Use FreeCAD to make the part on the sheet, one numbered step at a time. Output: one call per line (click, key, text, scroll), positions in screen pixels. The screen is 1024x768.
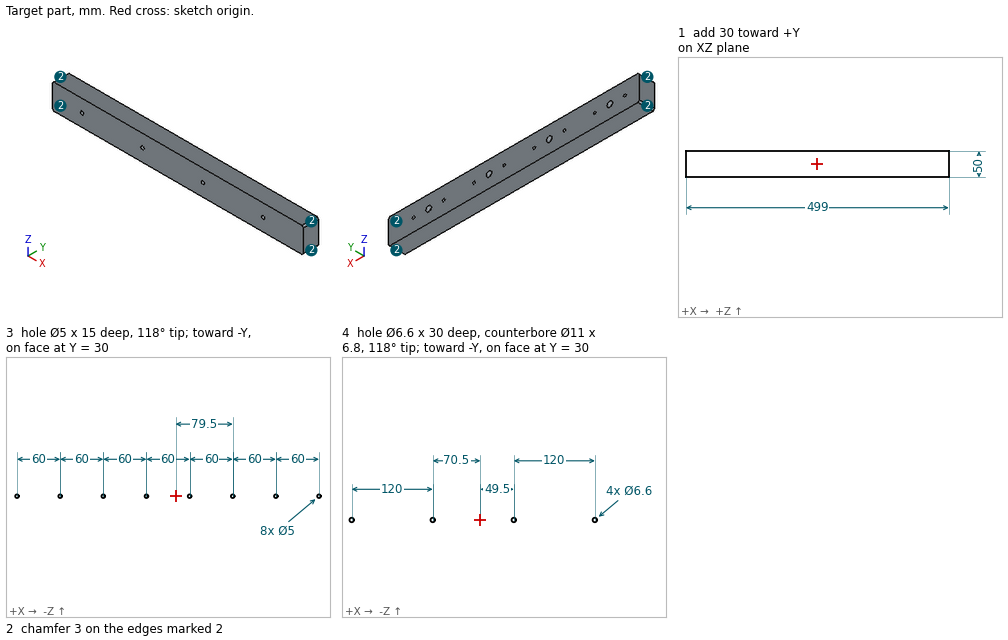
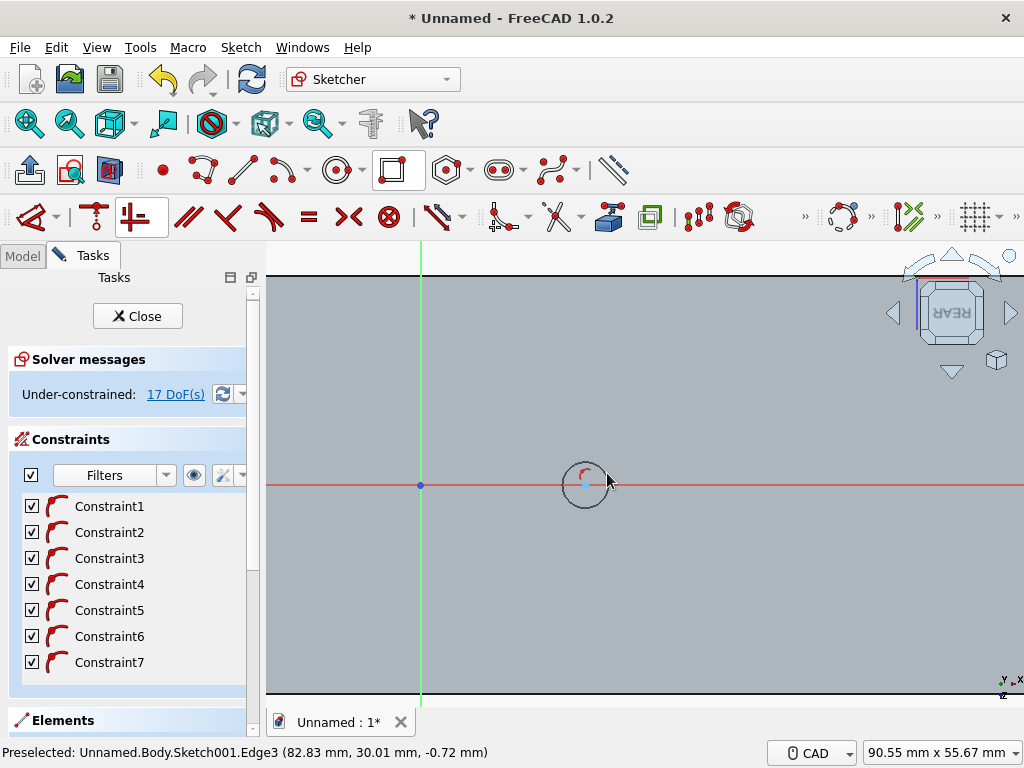
click(601, 469)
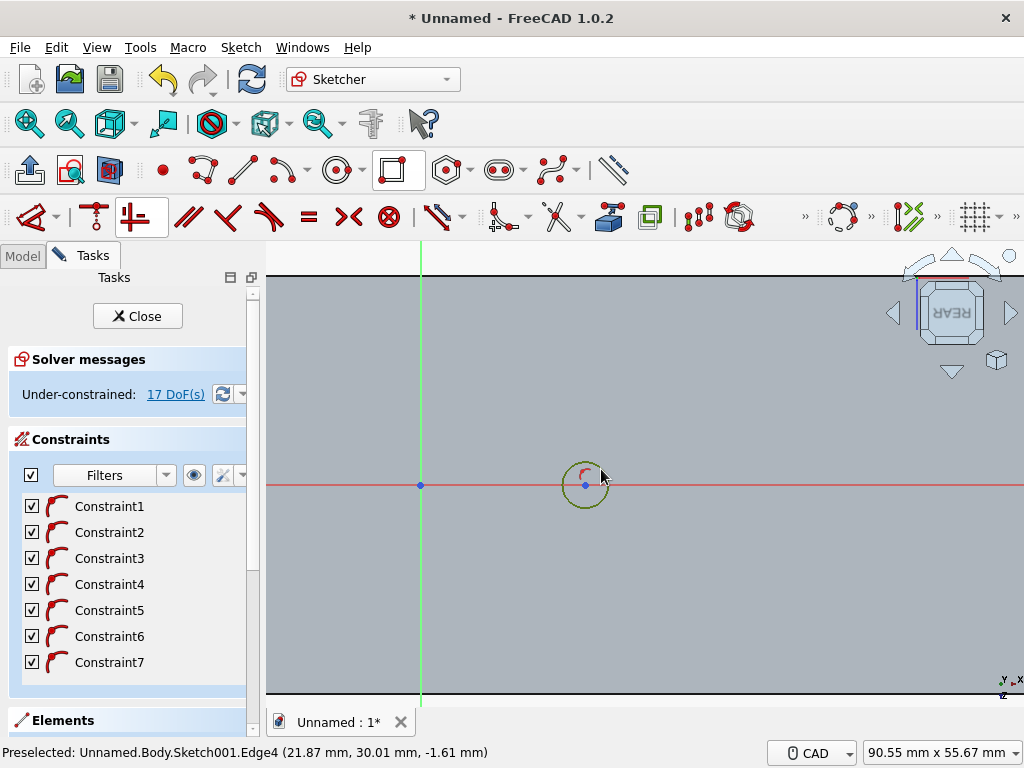
scroll(607, 473, down, 11)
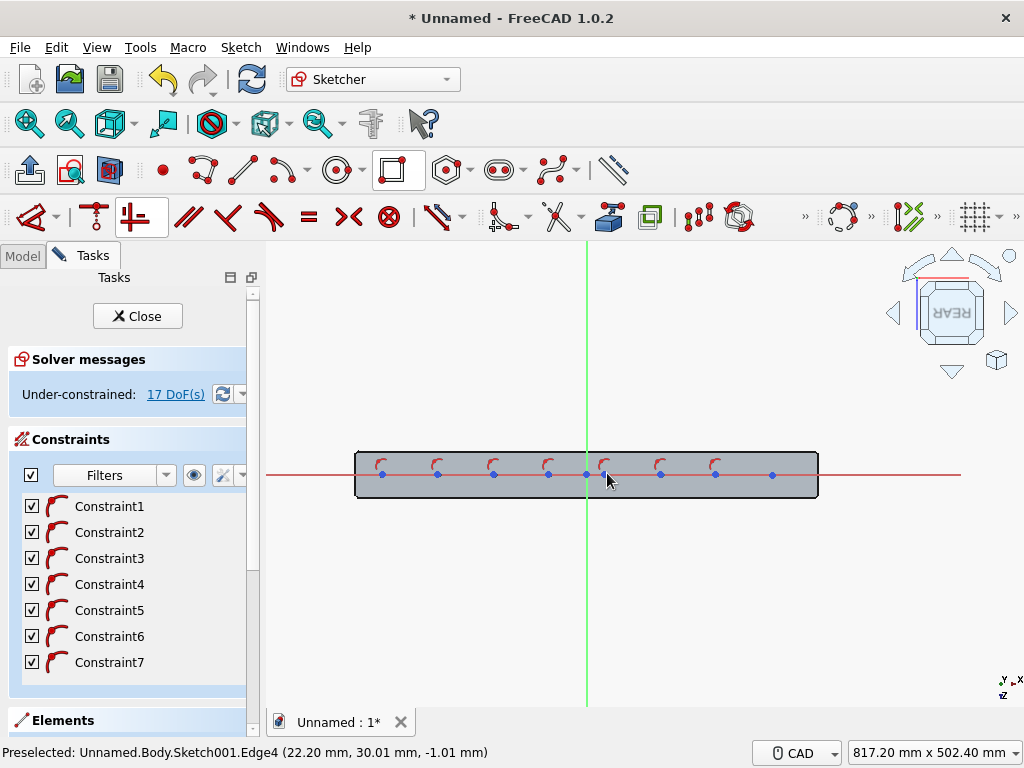
scroll(551, 473, up, 11)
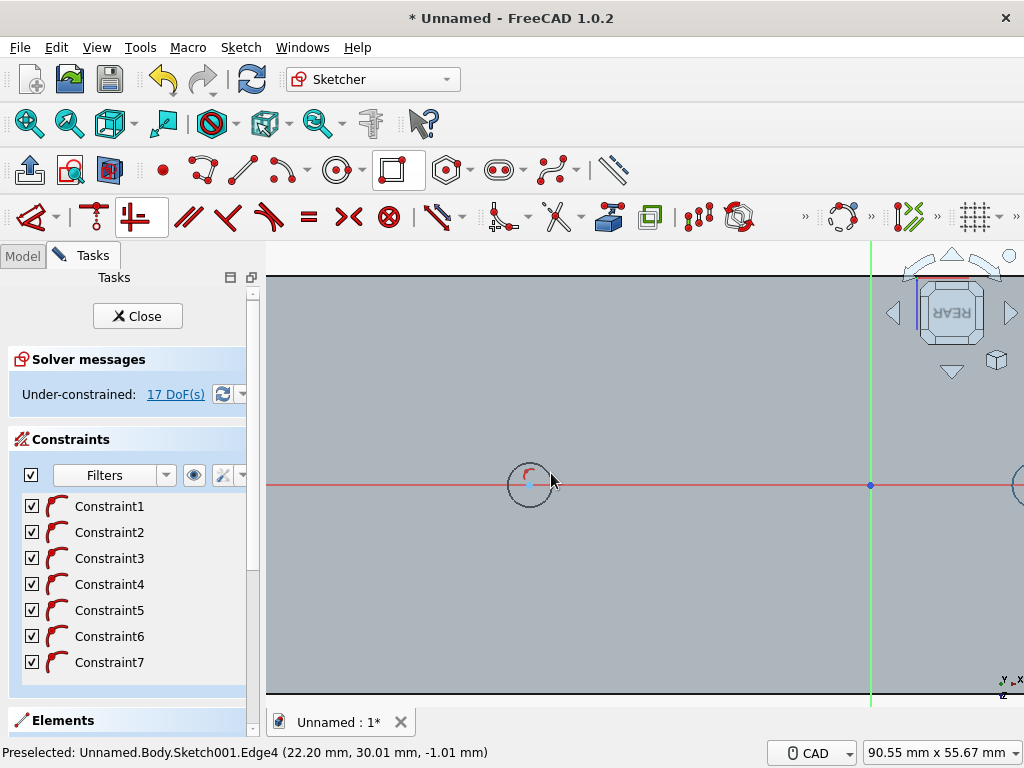
click(545, 470)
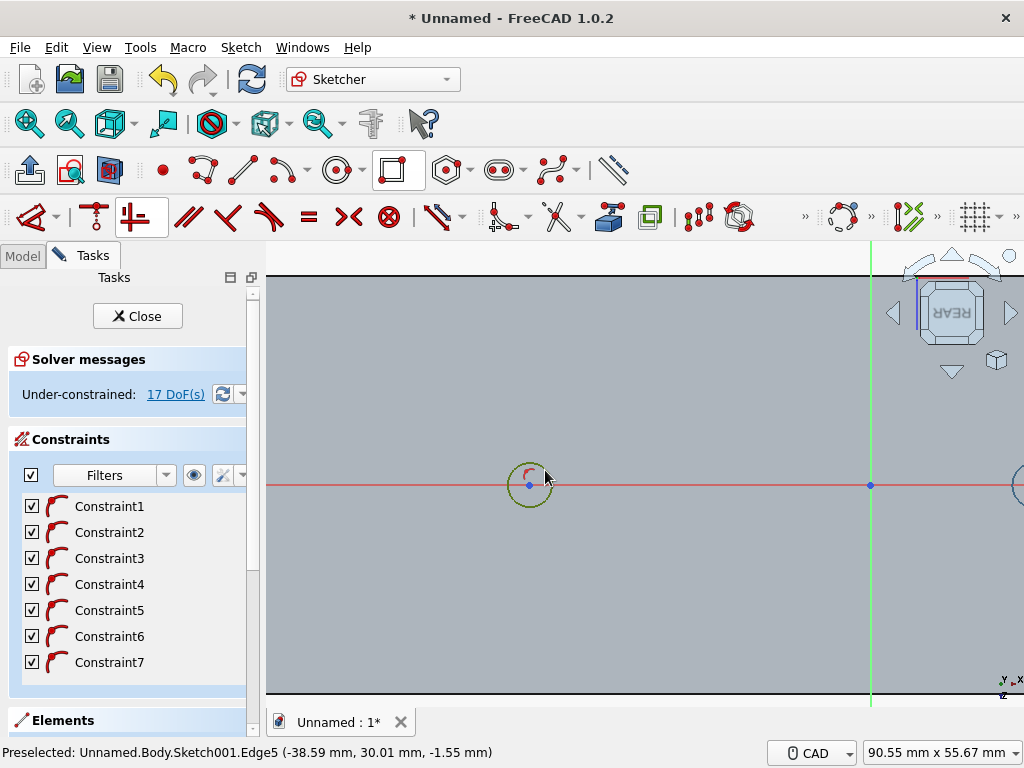
scroll(551, 473, down, 11)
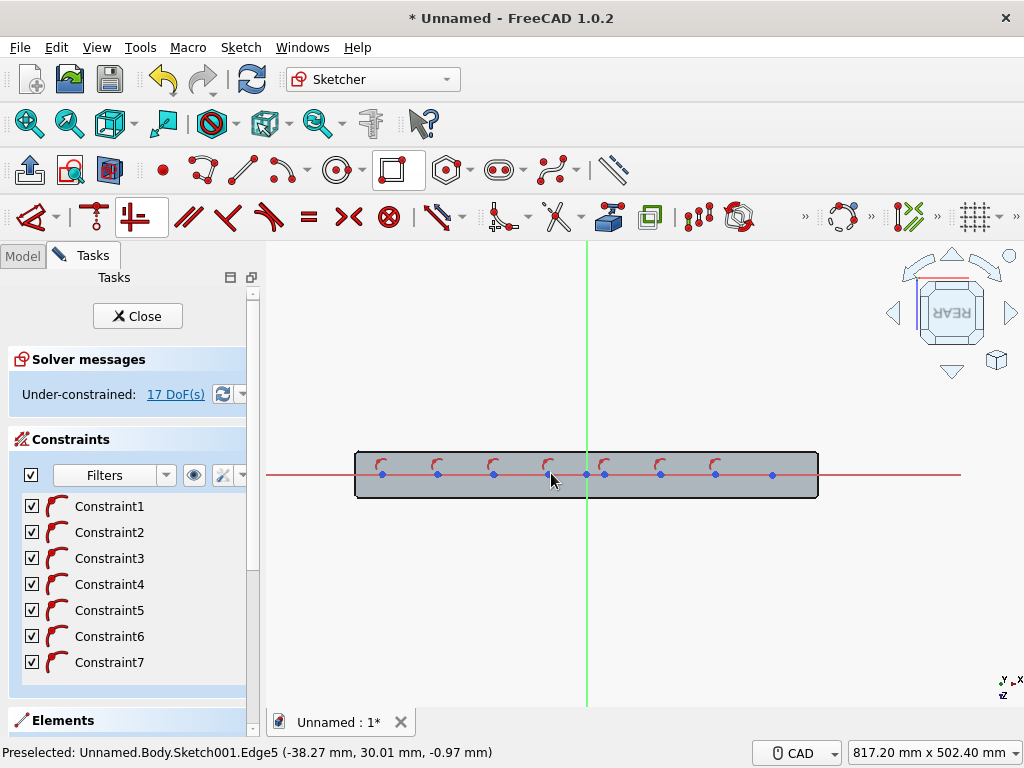
scroll(496, 473, up, 10)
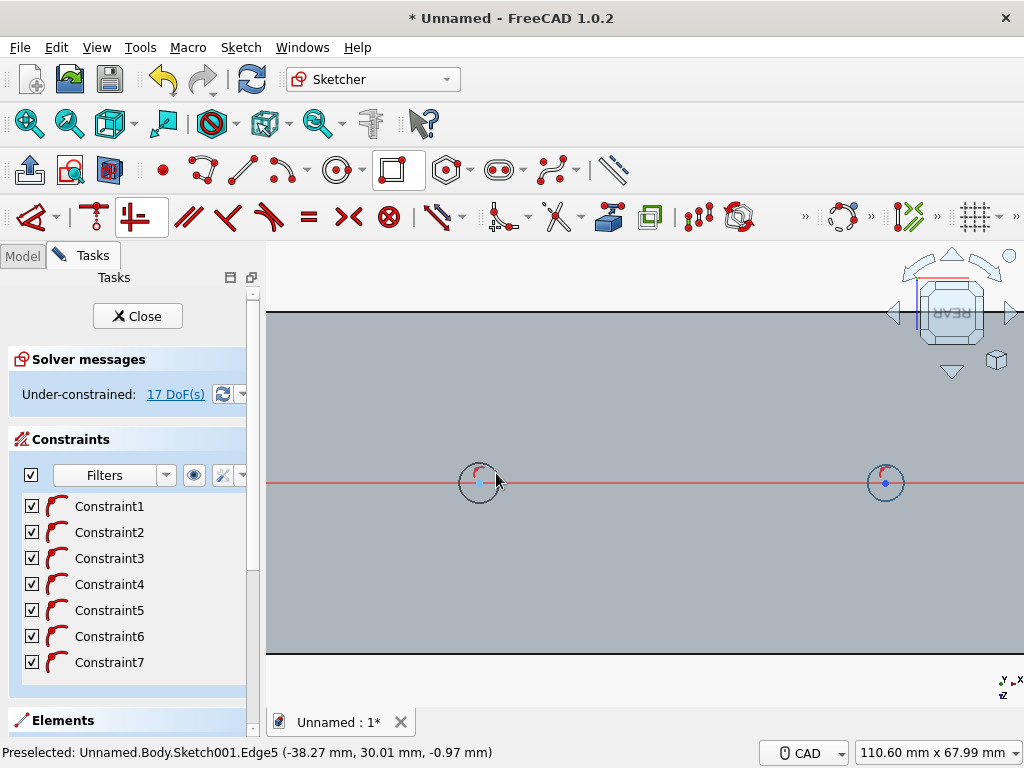
click(493, 469)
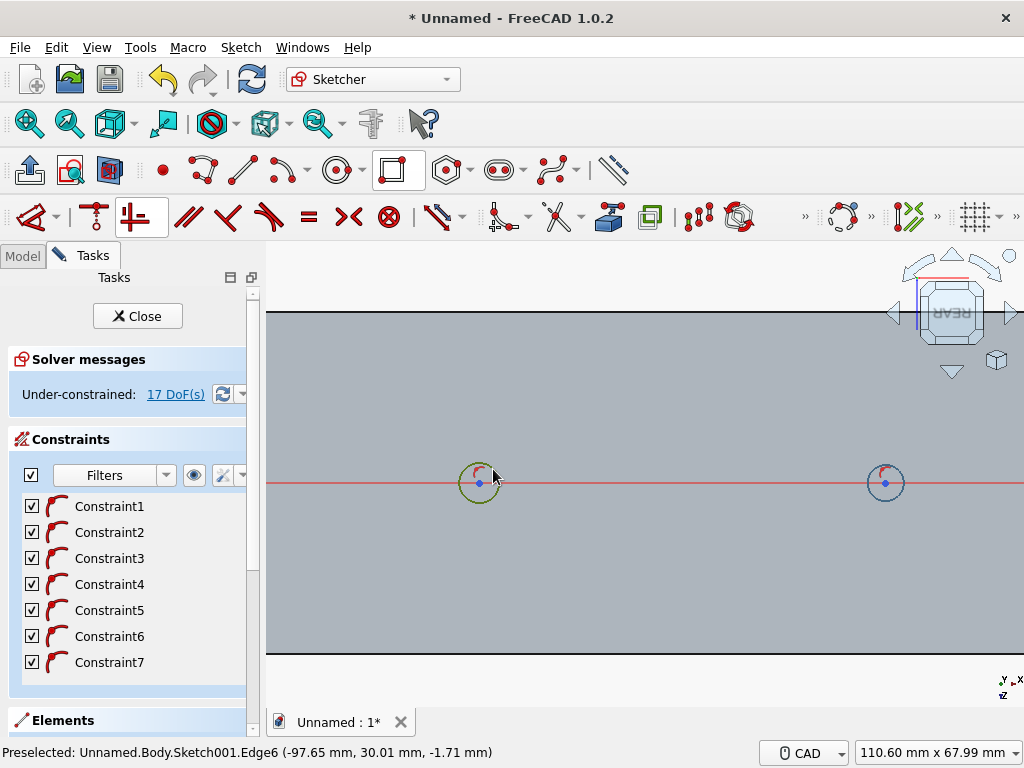
scroll(496, 473, down, 10)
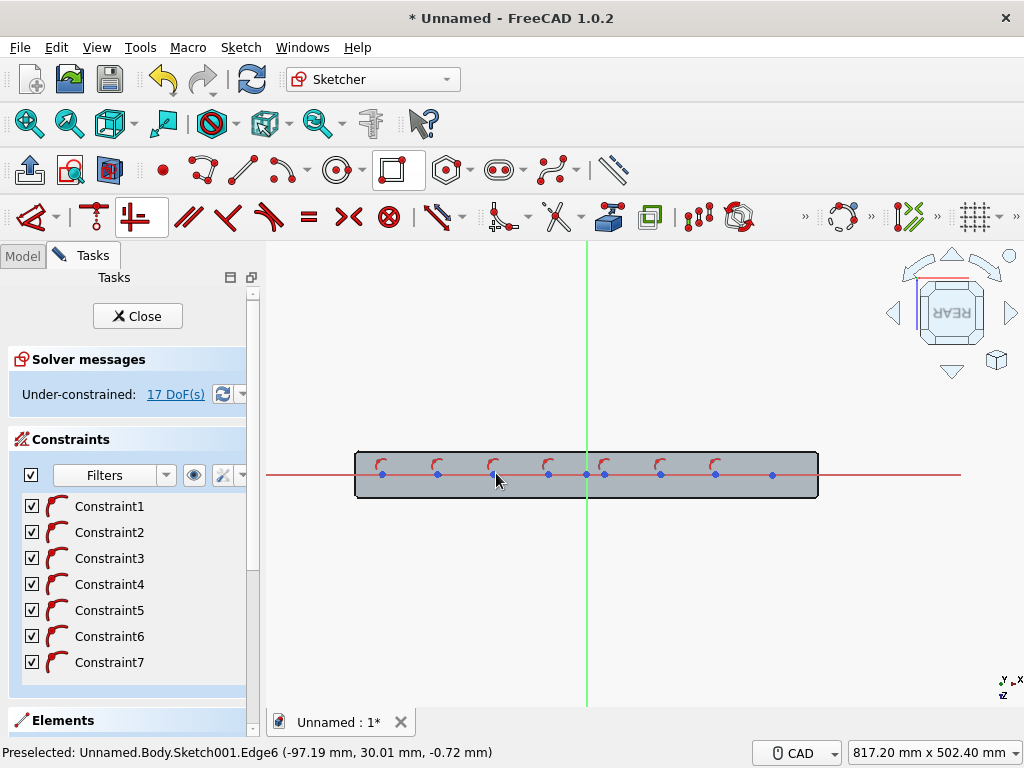
scroll(440, 473, up, 11)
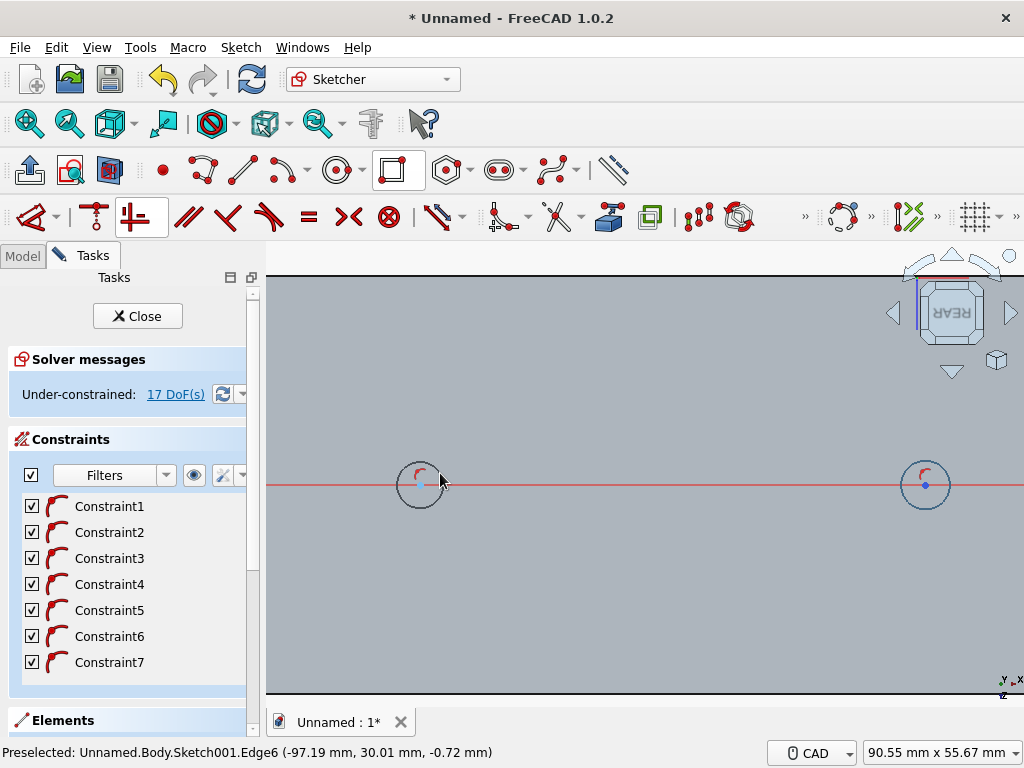
click(436, 469)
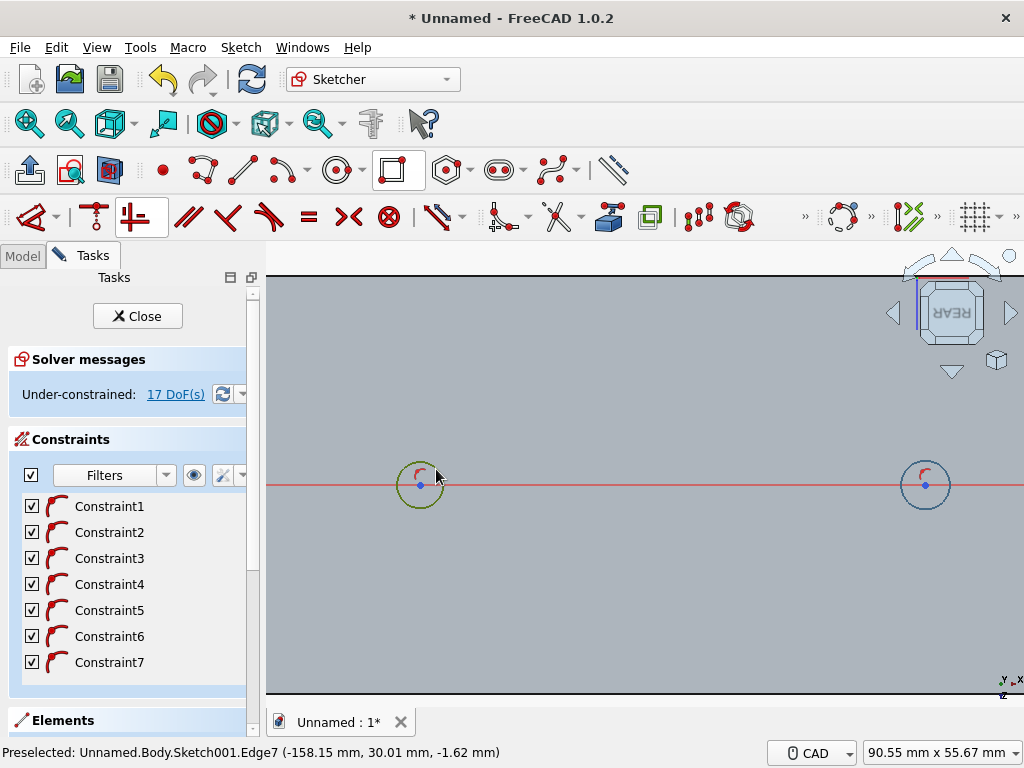
scroll(440, 473, down, 11)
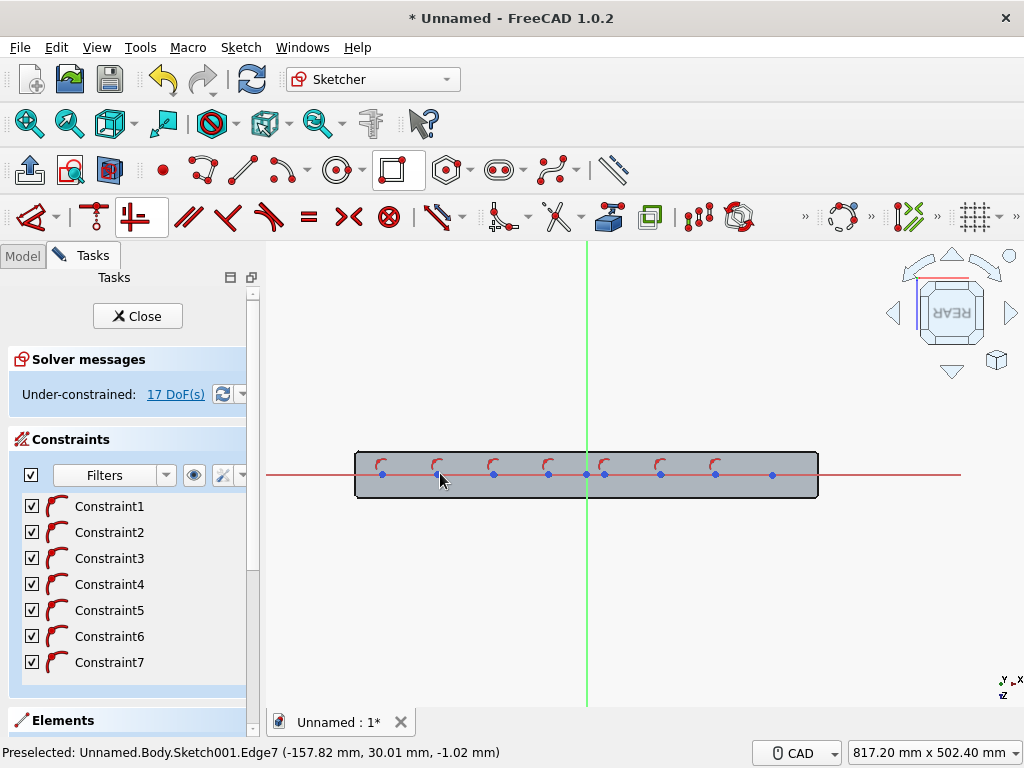
scroll(384, 473, up, 11)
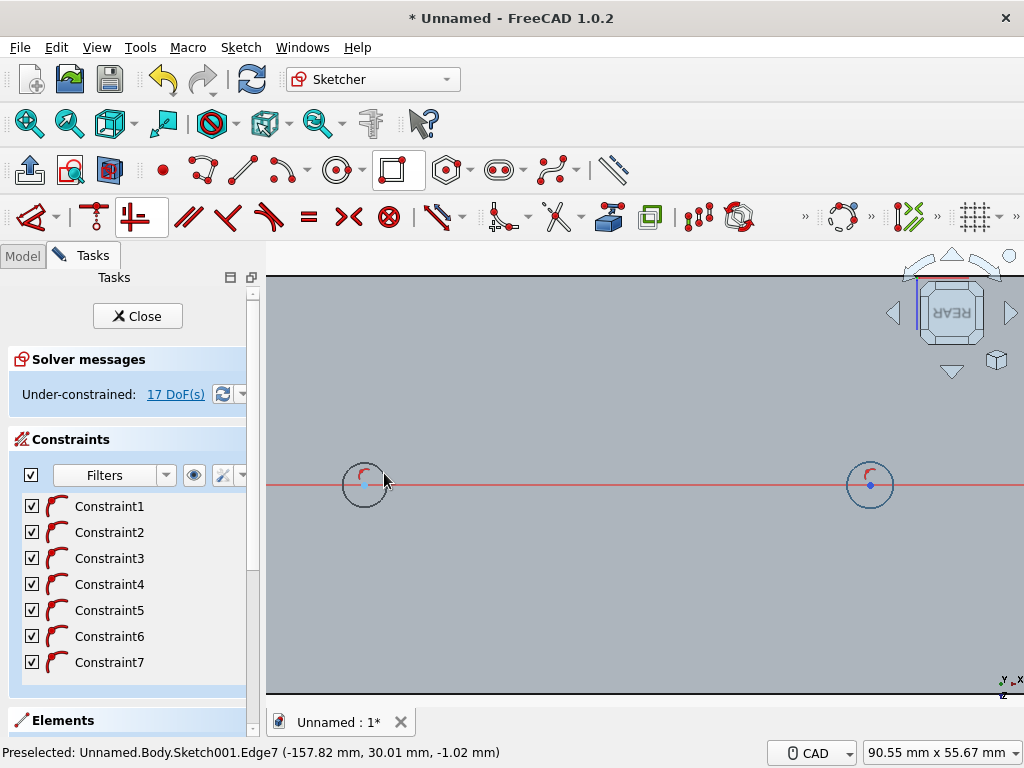
click(380, 469)